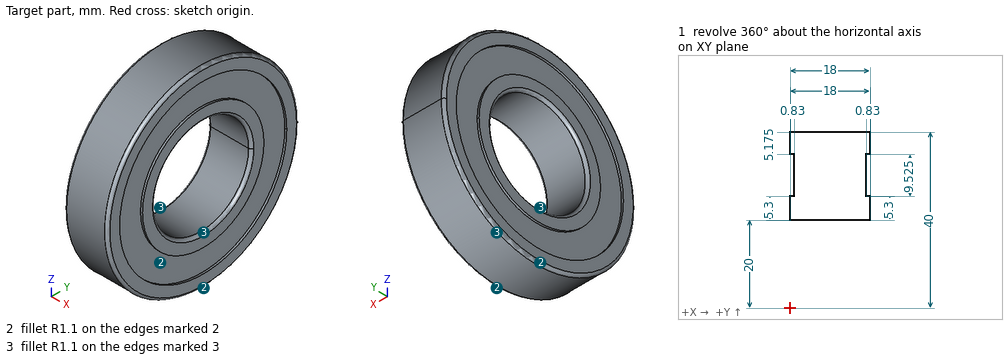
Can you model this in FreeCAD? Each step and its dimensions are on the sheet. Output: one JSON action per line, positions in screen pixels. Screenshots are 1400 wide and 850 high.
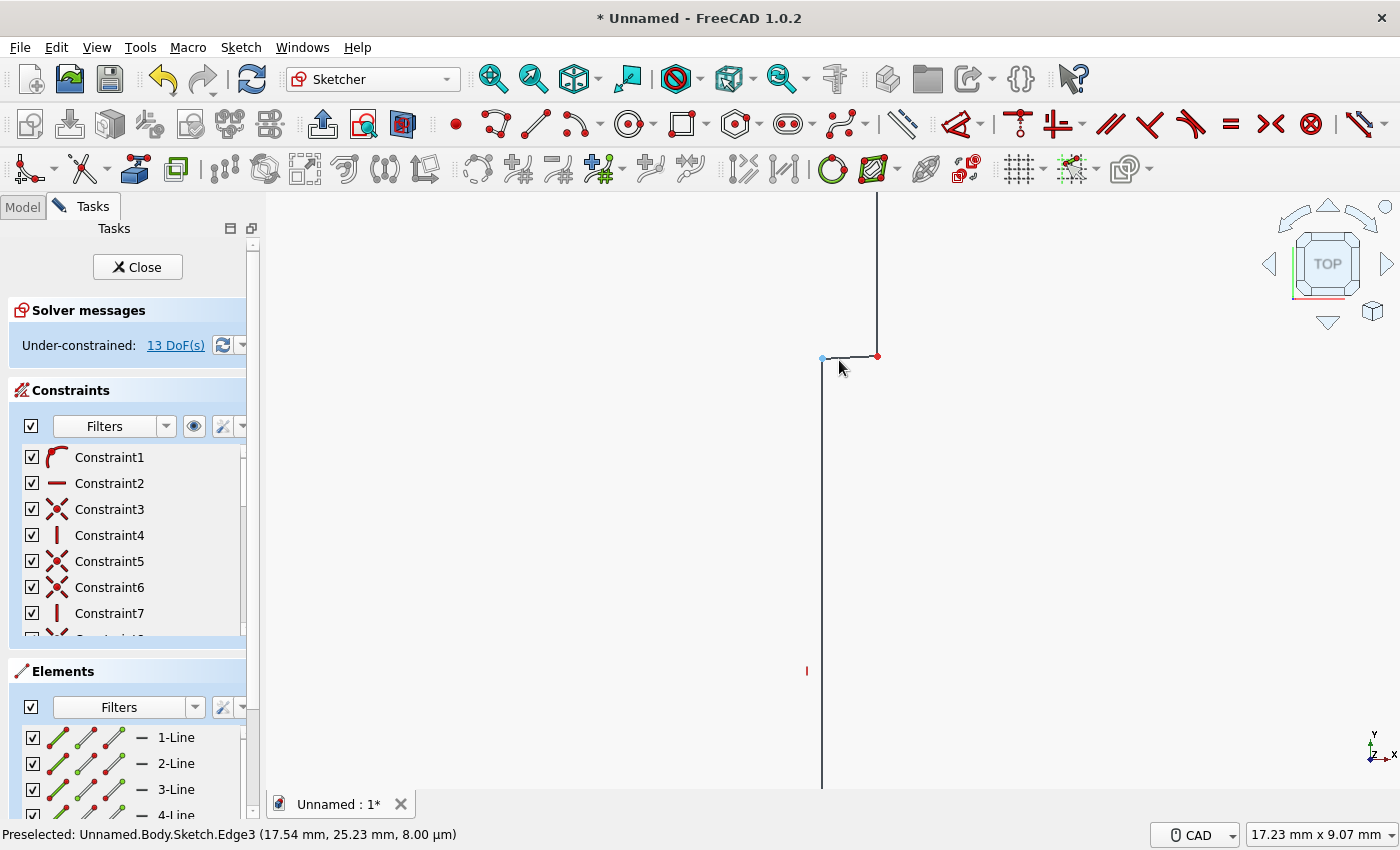
{"action": "left_click", "coordinate": [839, 358]}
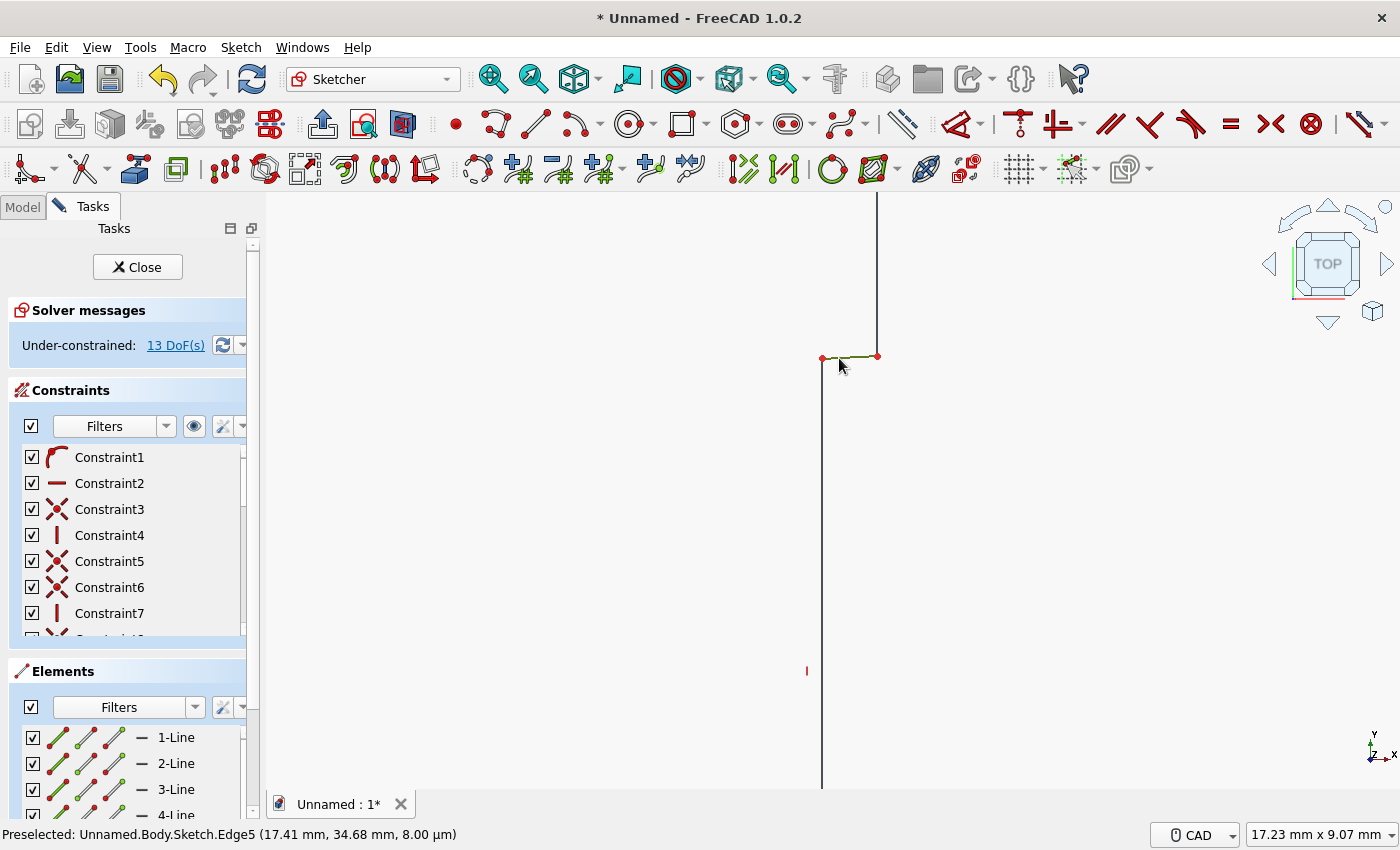
{"action": "left_click", "coordinate": [1084, 124]}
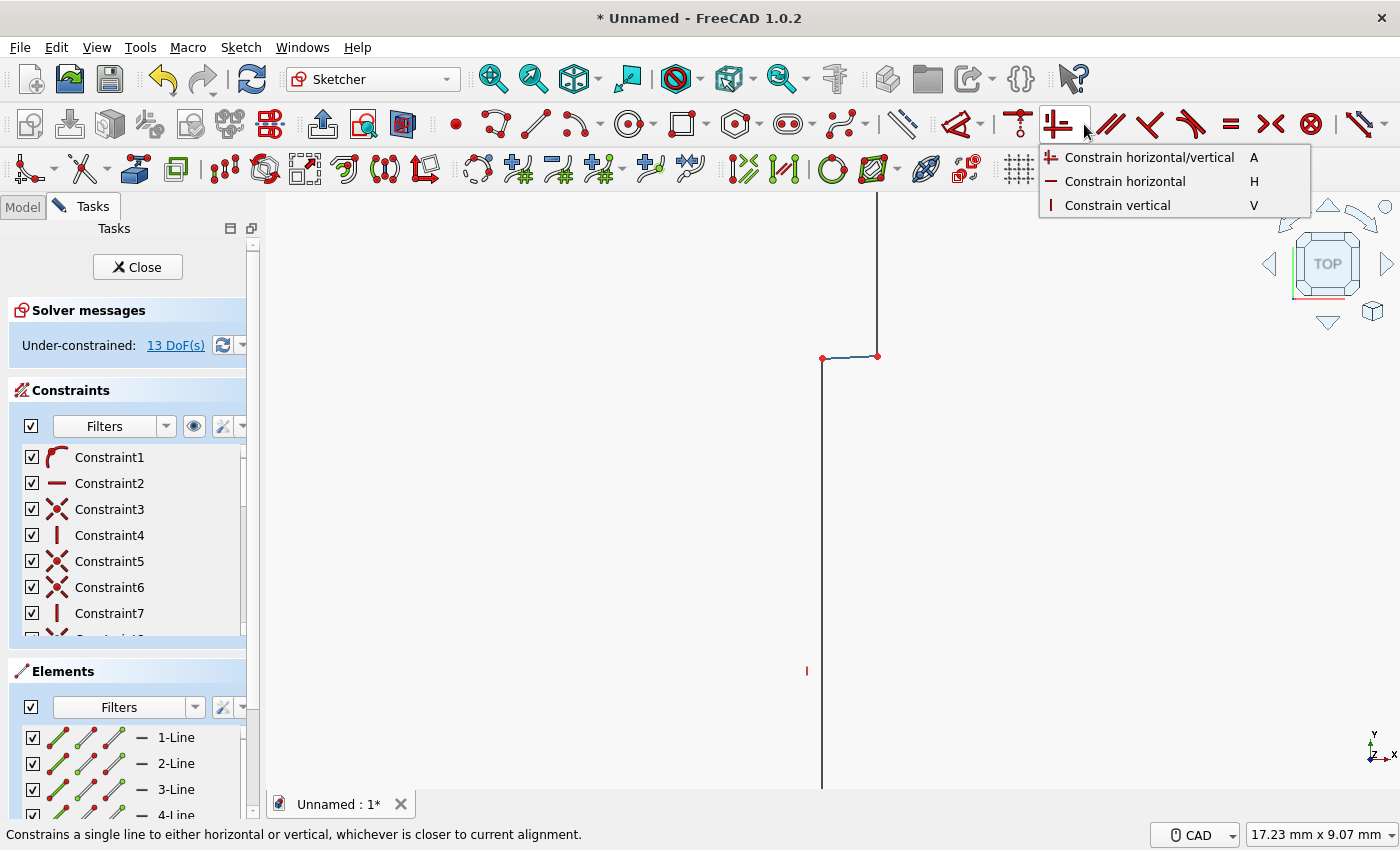
{"action": "left_click", "coordinate": [1175, 181]}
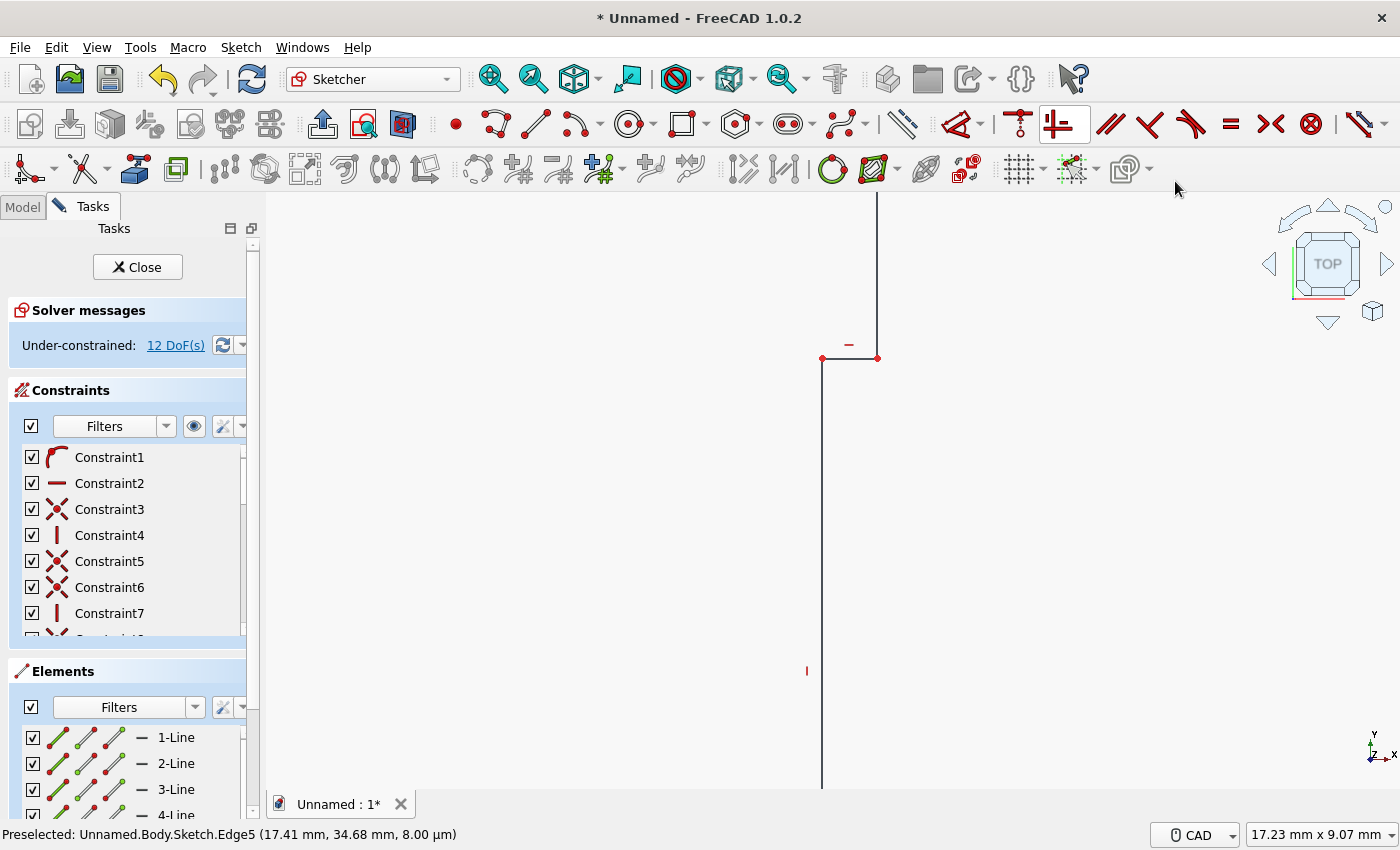
{"action": "scroll", "coordinate": [839, 360], "scroll_direction": "down", "scroll_amount": 10}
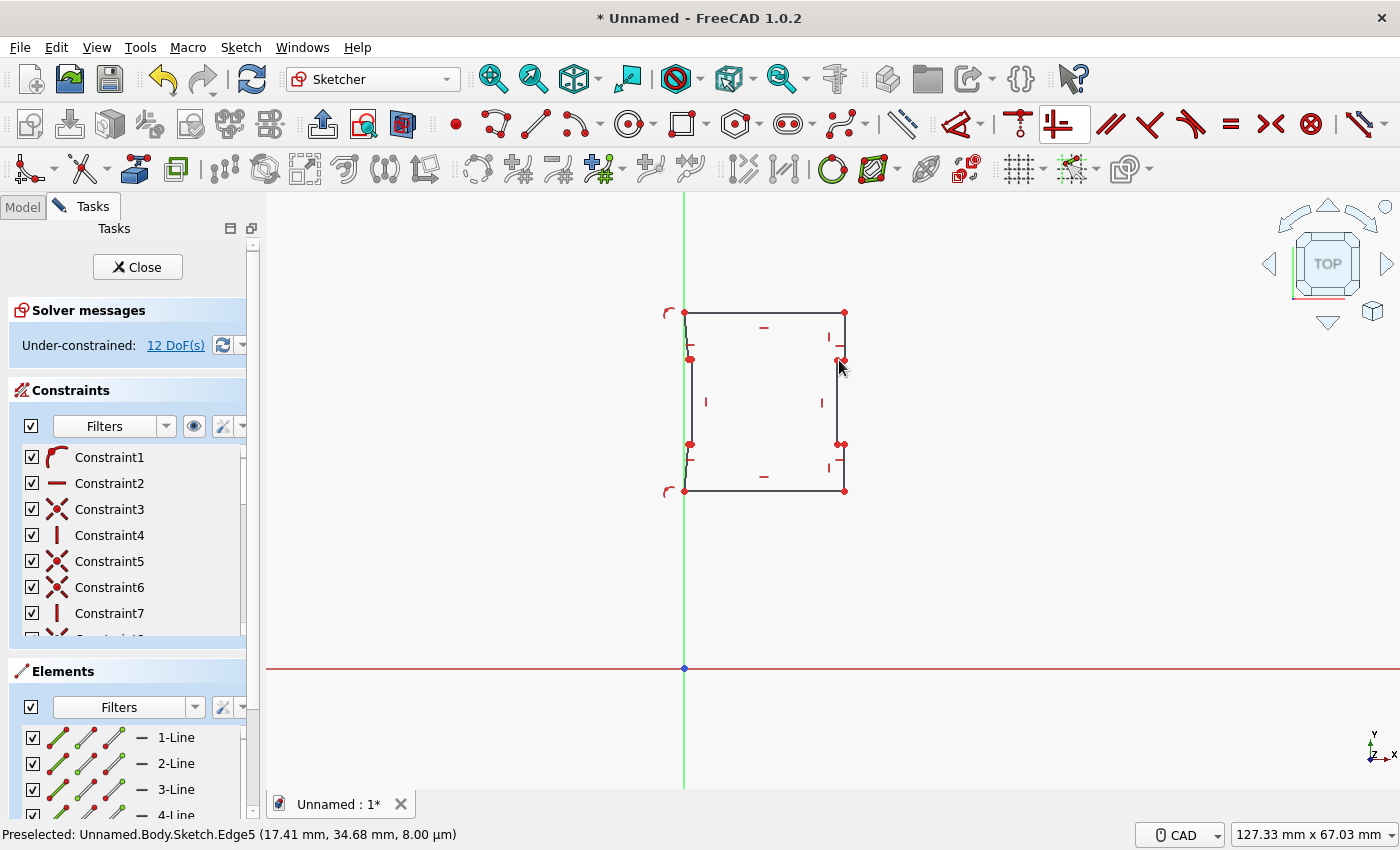
{"action": "scroll", "coordinate": [687, 345], "scroll_direction": "up", "scroll_amount": 9}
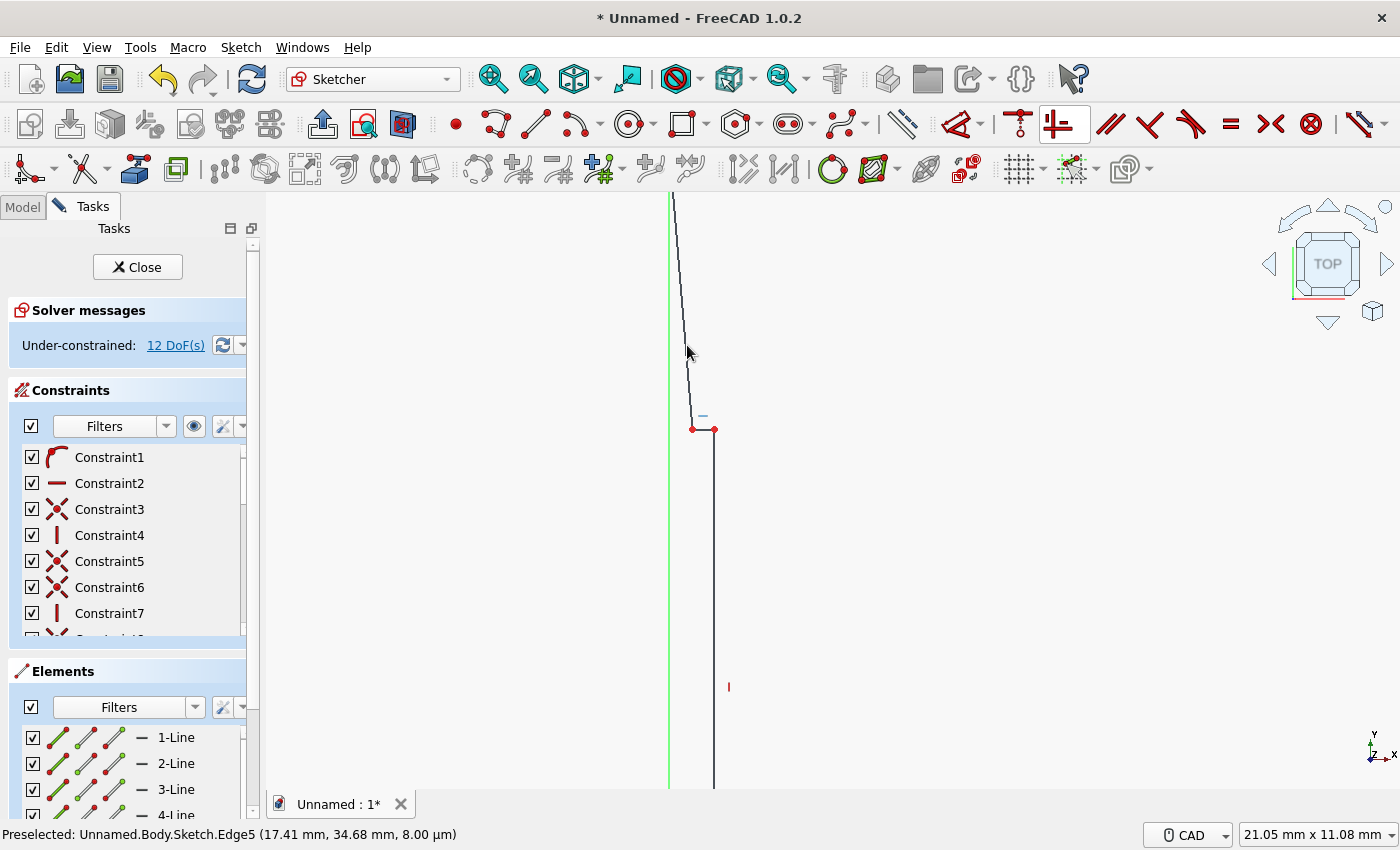
{"action": "left_click", "coordinate": [686, 346]}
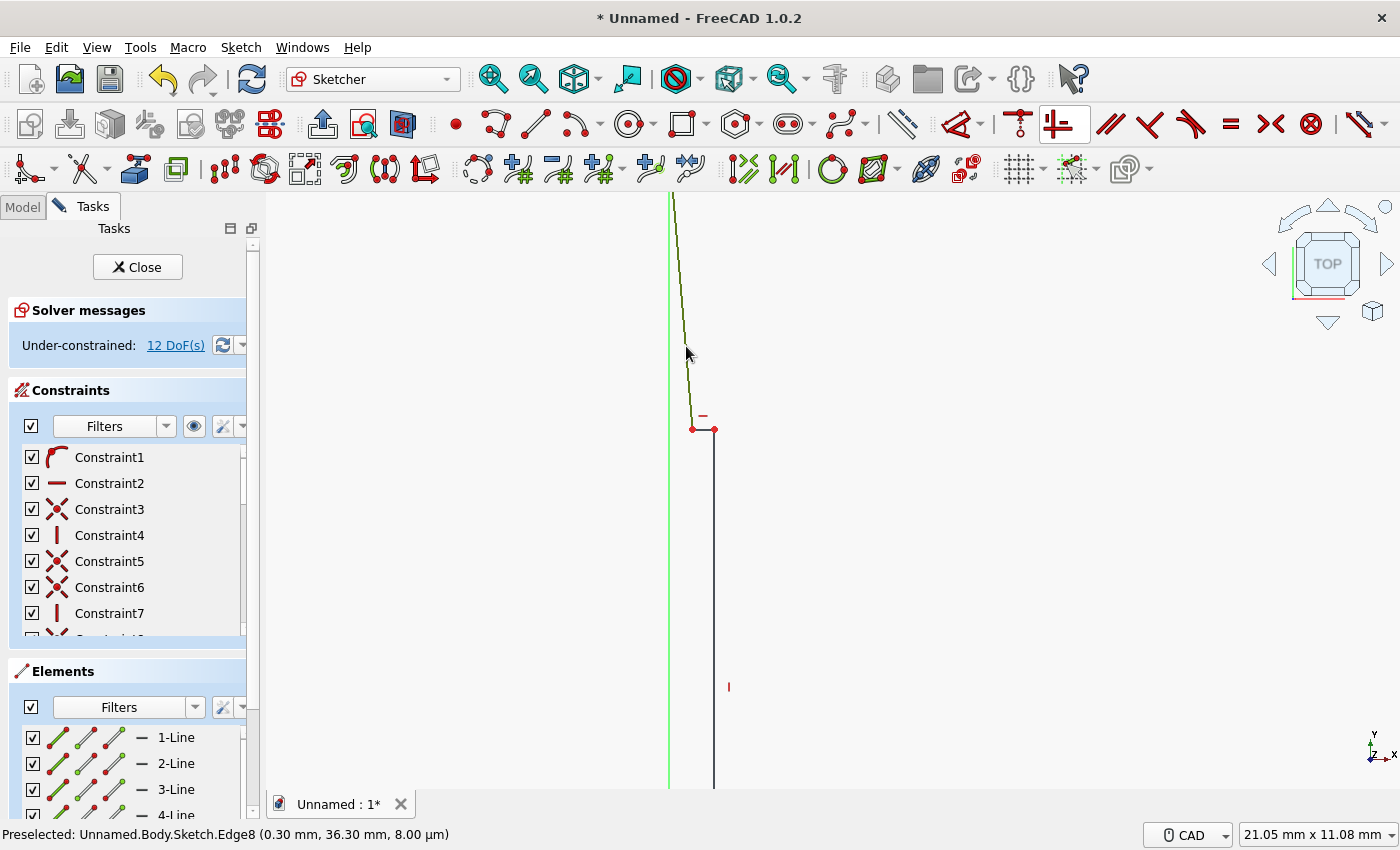
{"action": "key", "text": "v"}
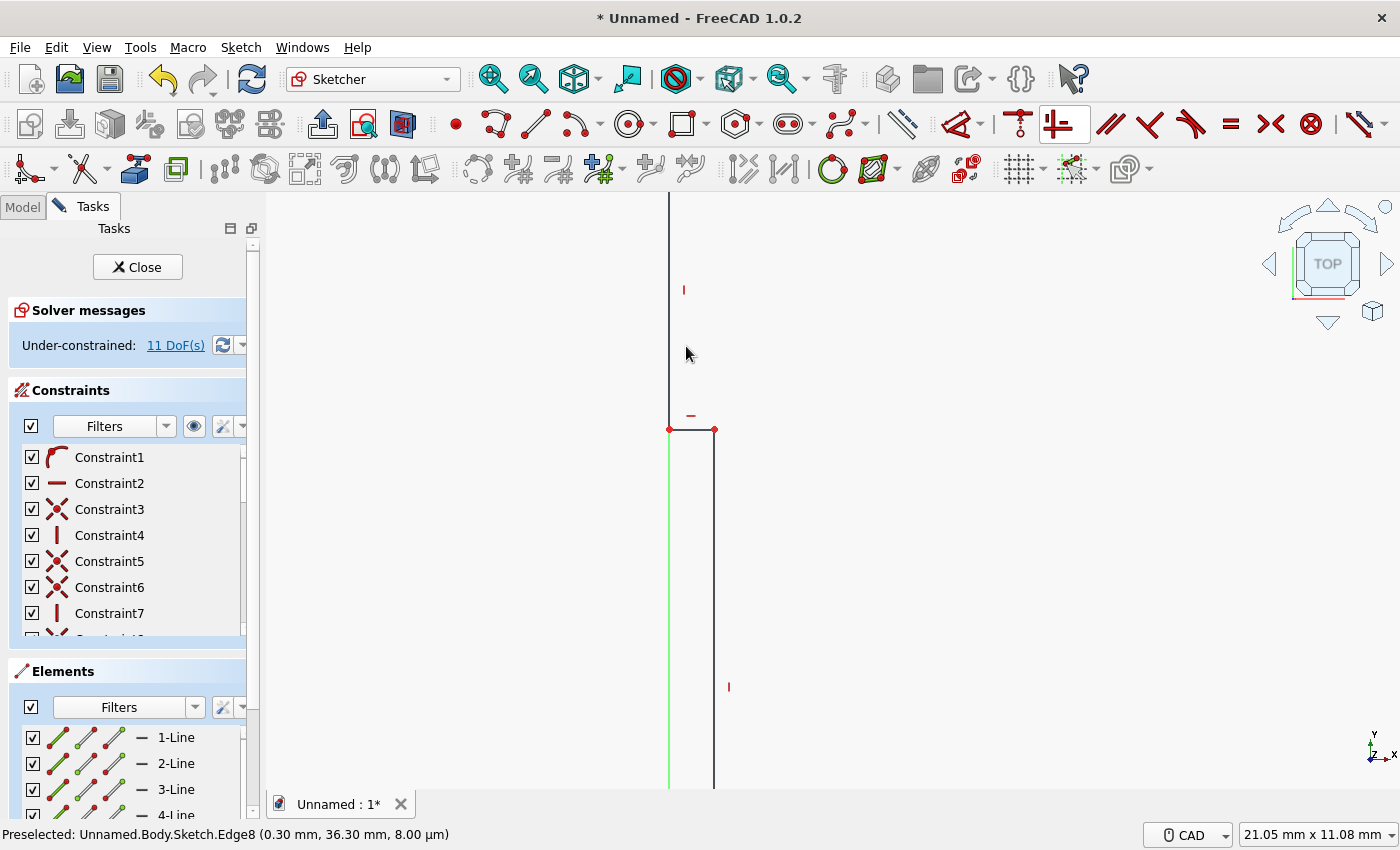
{"action": "scroll", "coordinate": [687, 345], "scroll_direction": "down", "scroll_amount": 9}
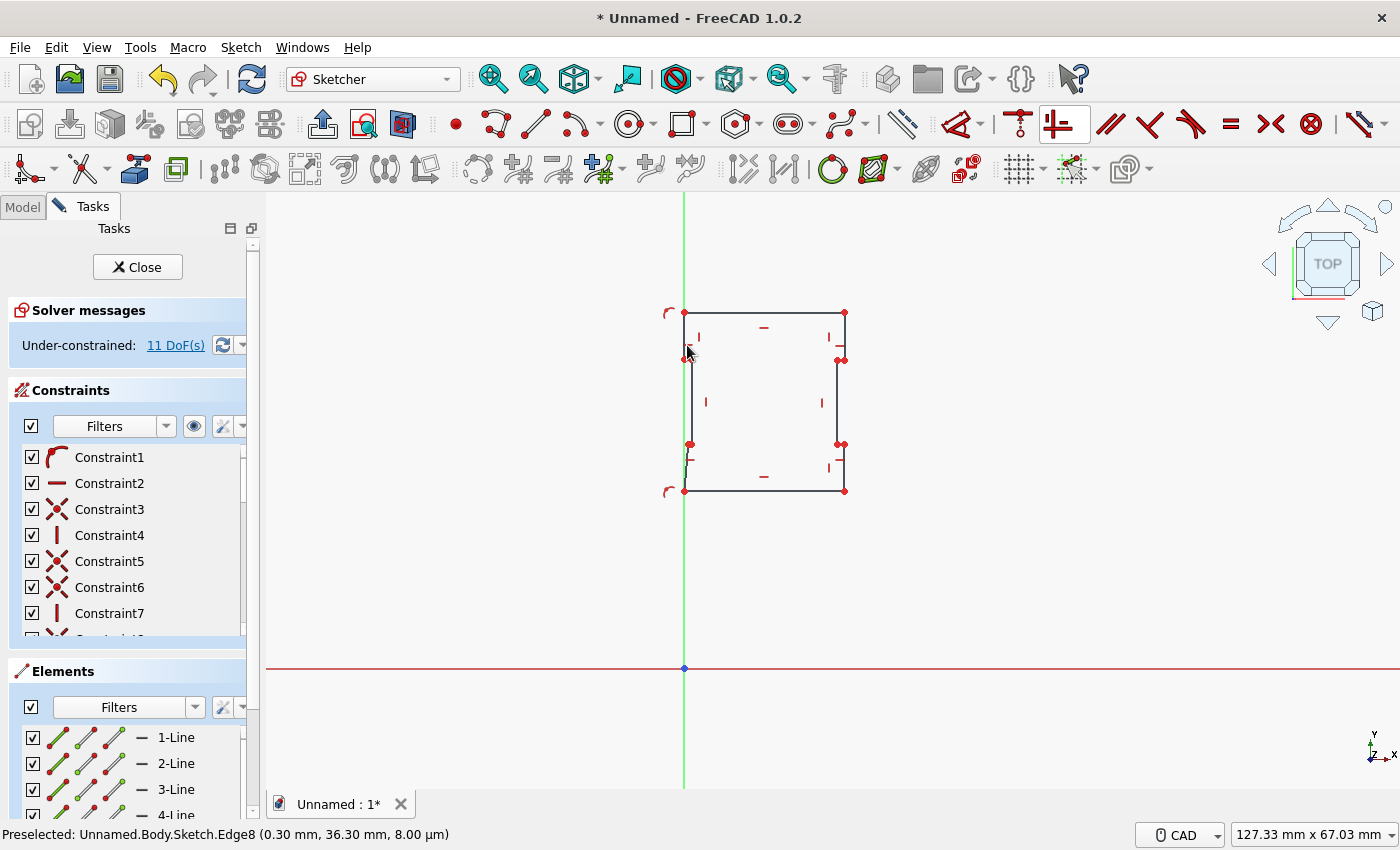
{"action": "scroll", "coordinate": [687, 458], "scroll_direction": "up", "scroll_amount": 9}